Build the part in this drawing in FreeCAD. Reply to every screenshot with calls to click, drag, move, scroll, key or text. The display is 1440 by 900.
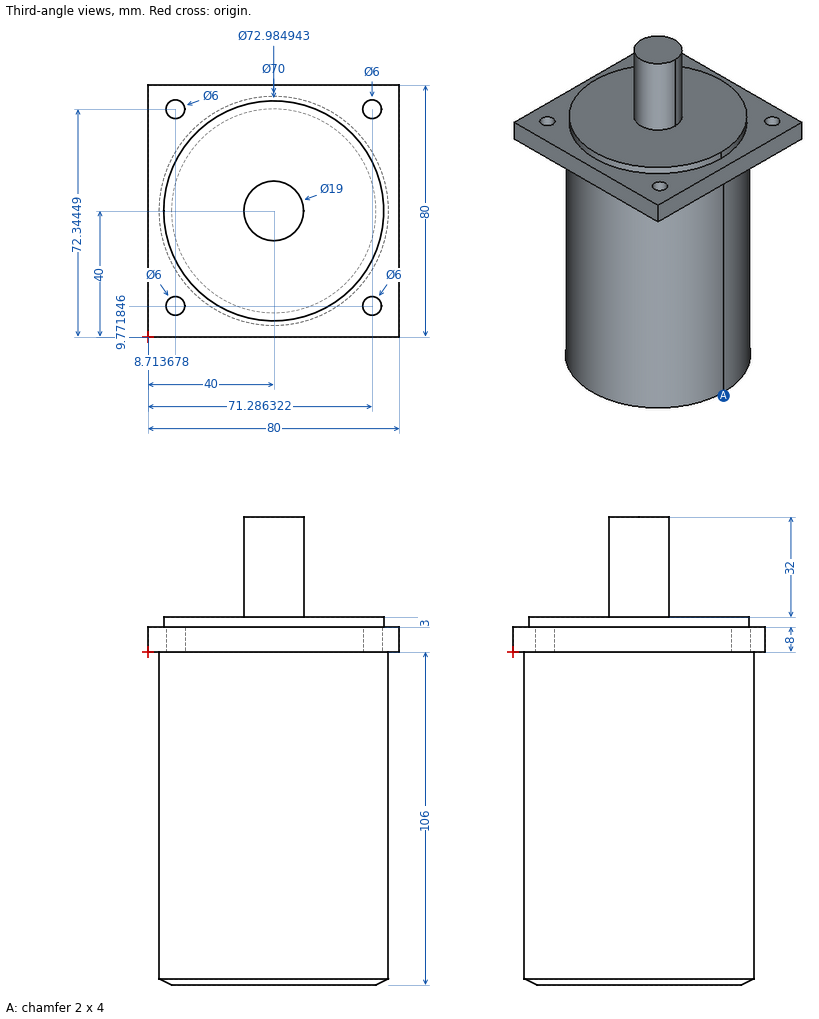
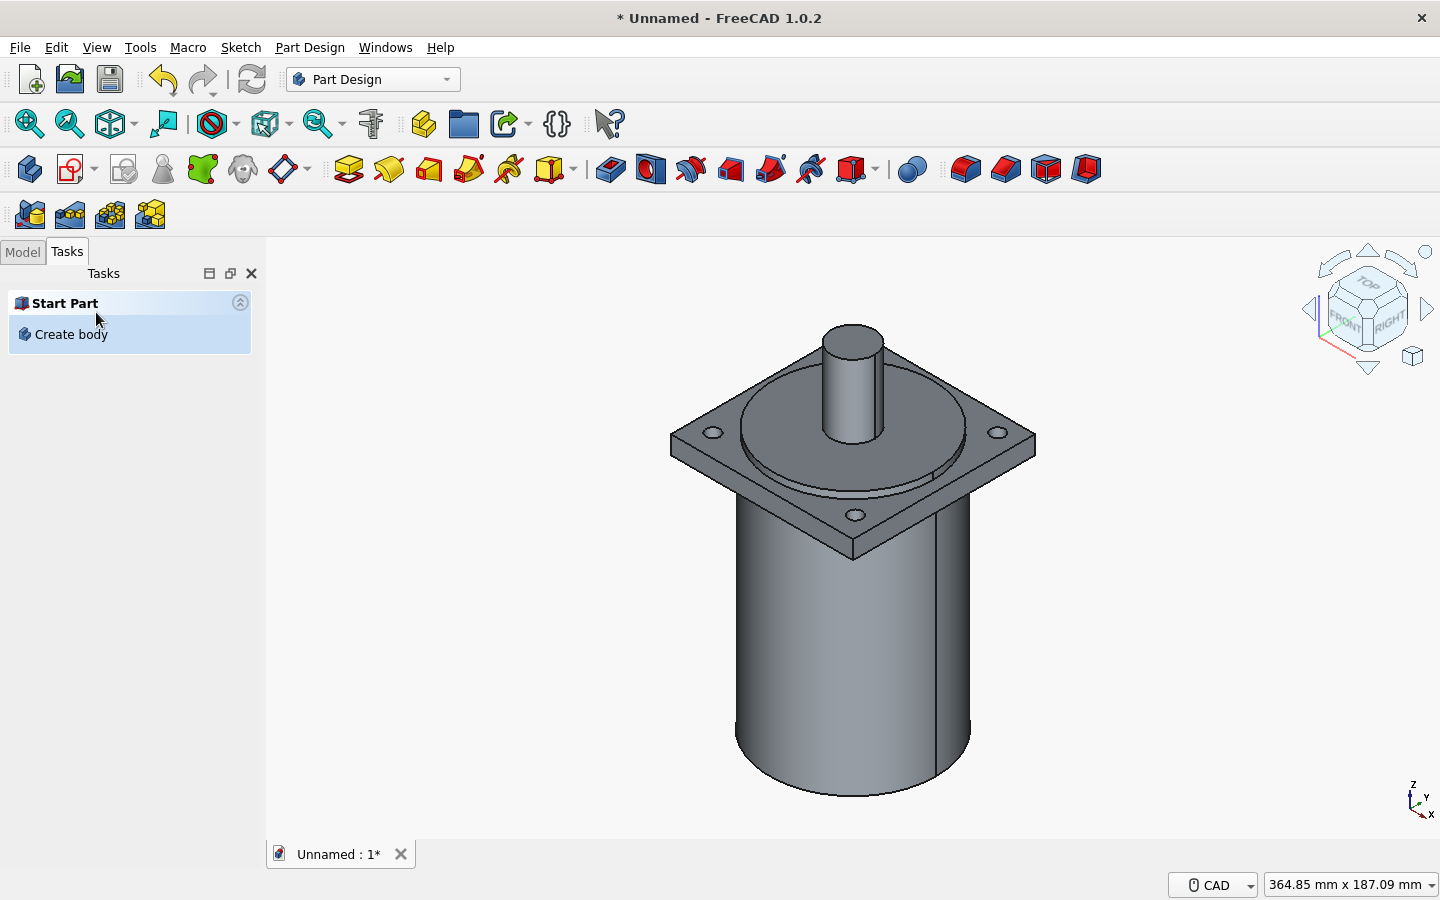
click(30, 124)